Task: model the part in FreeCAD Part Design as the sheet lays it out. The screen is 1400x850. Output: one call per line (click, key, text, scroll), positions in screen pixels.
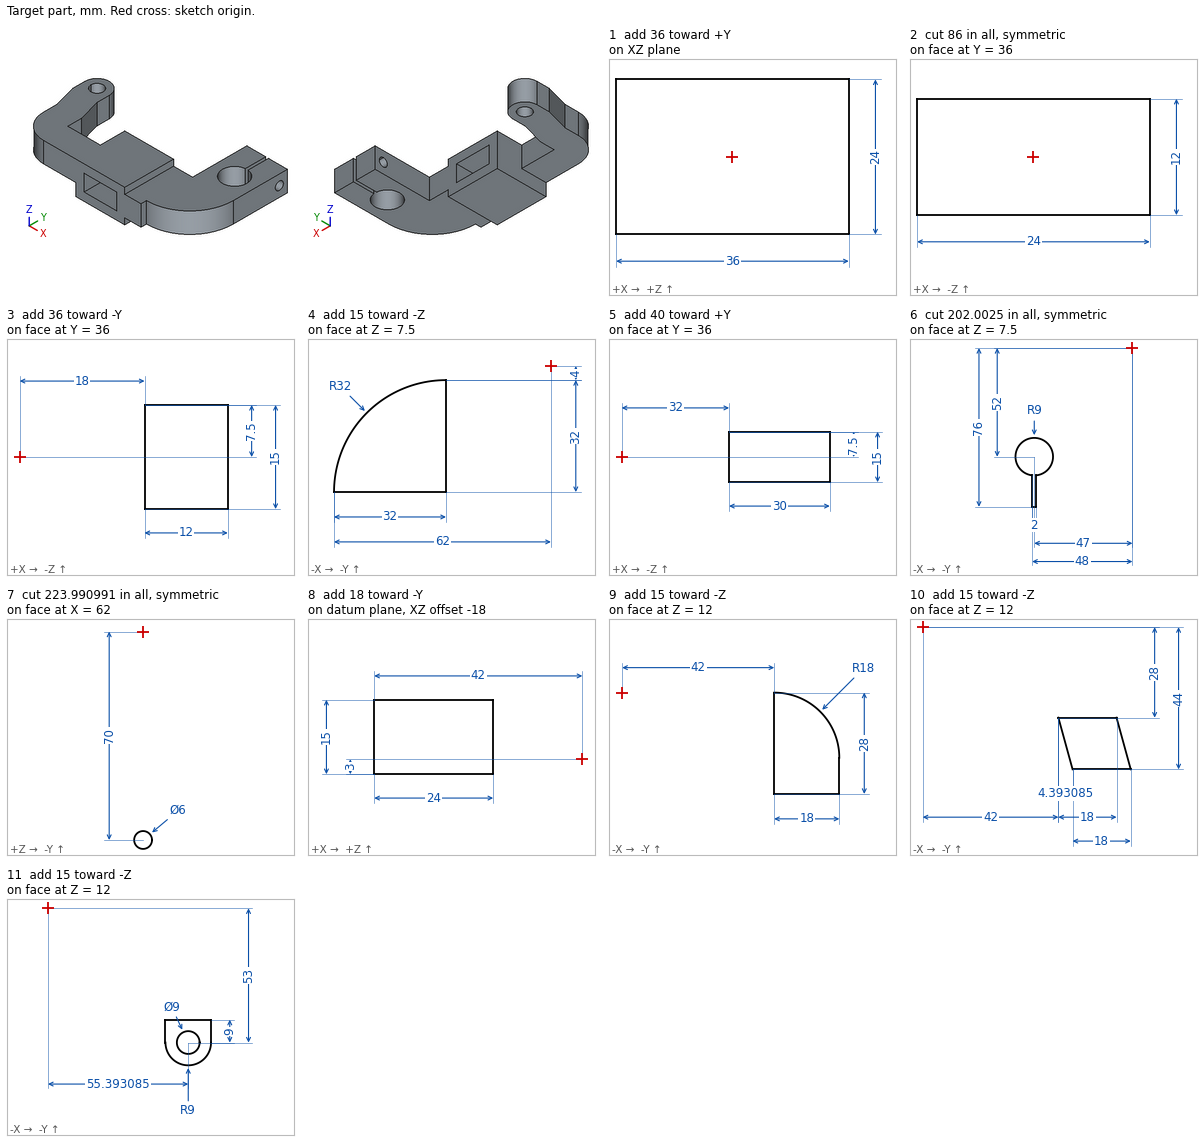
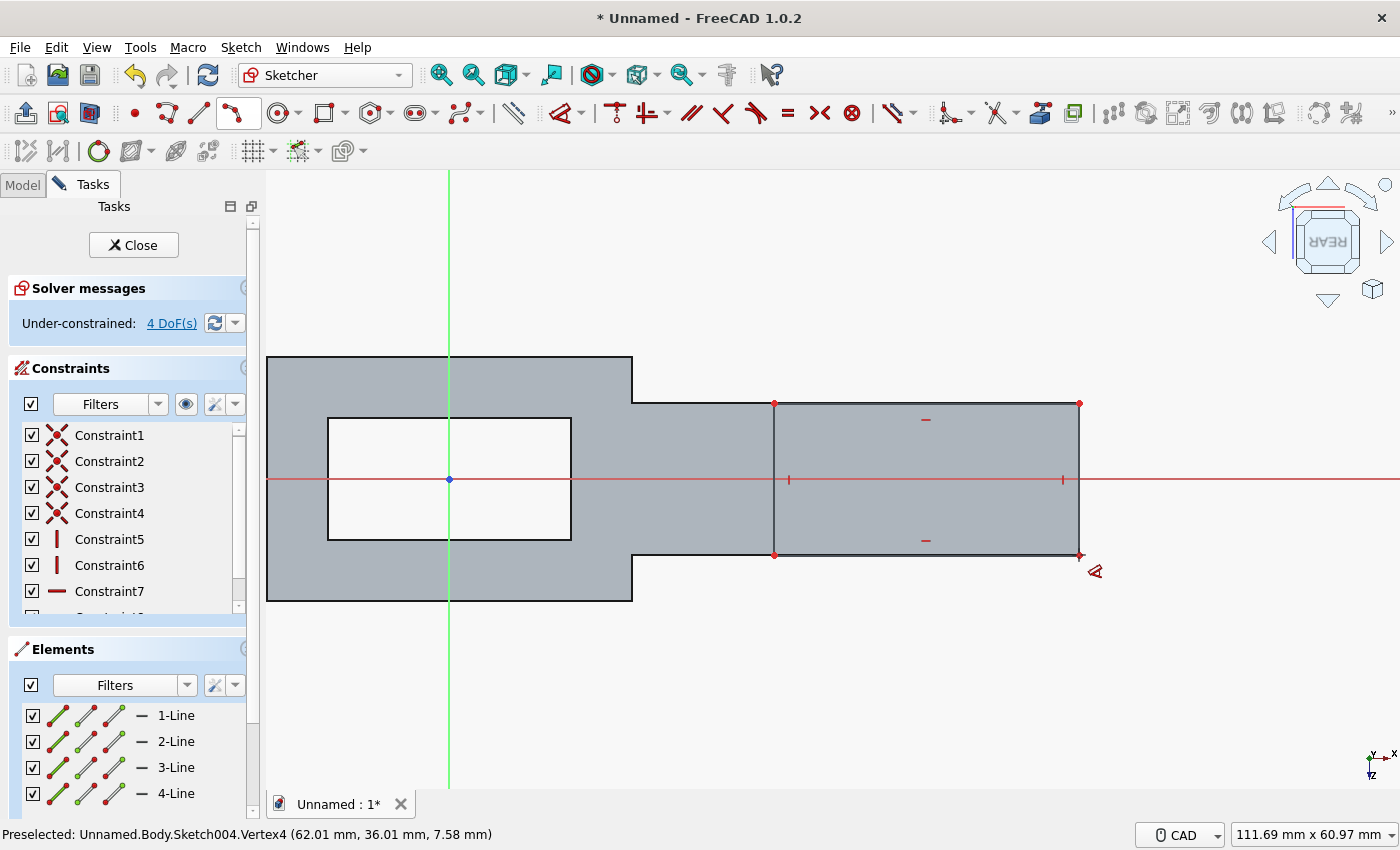
click(774, 450)
click(808, 445)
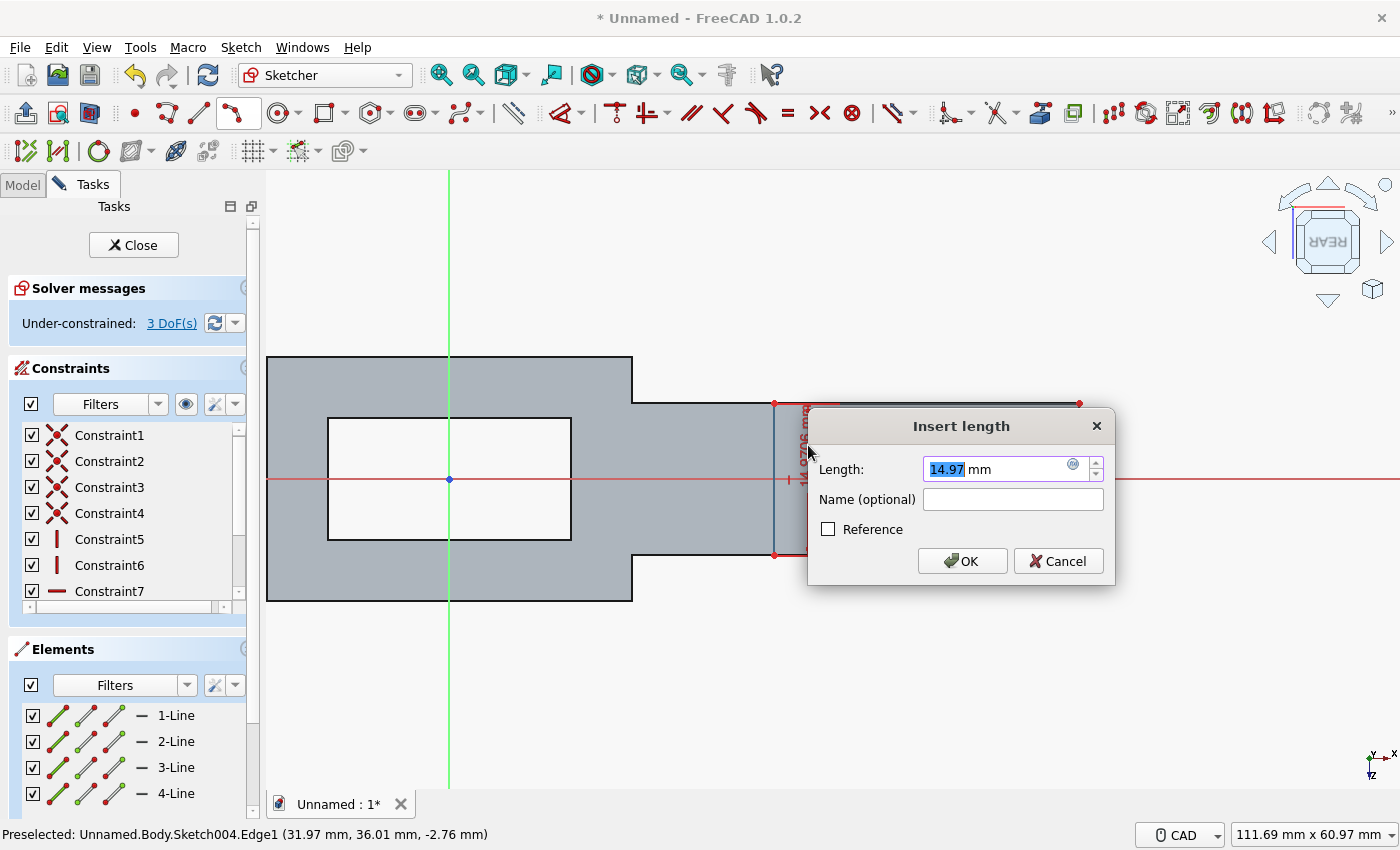
text(15)
key(Return)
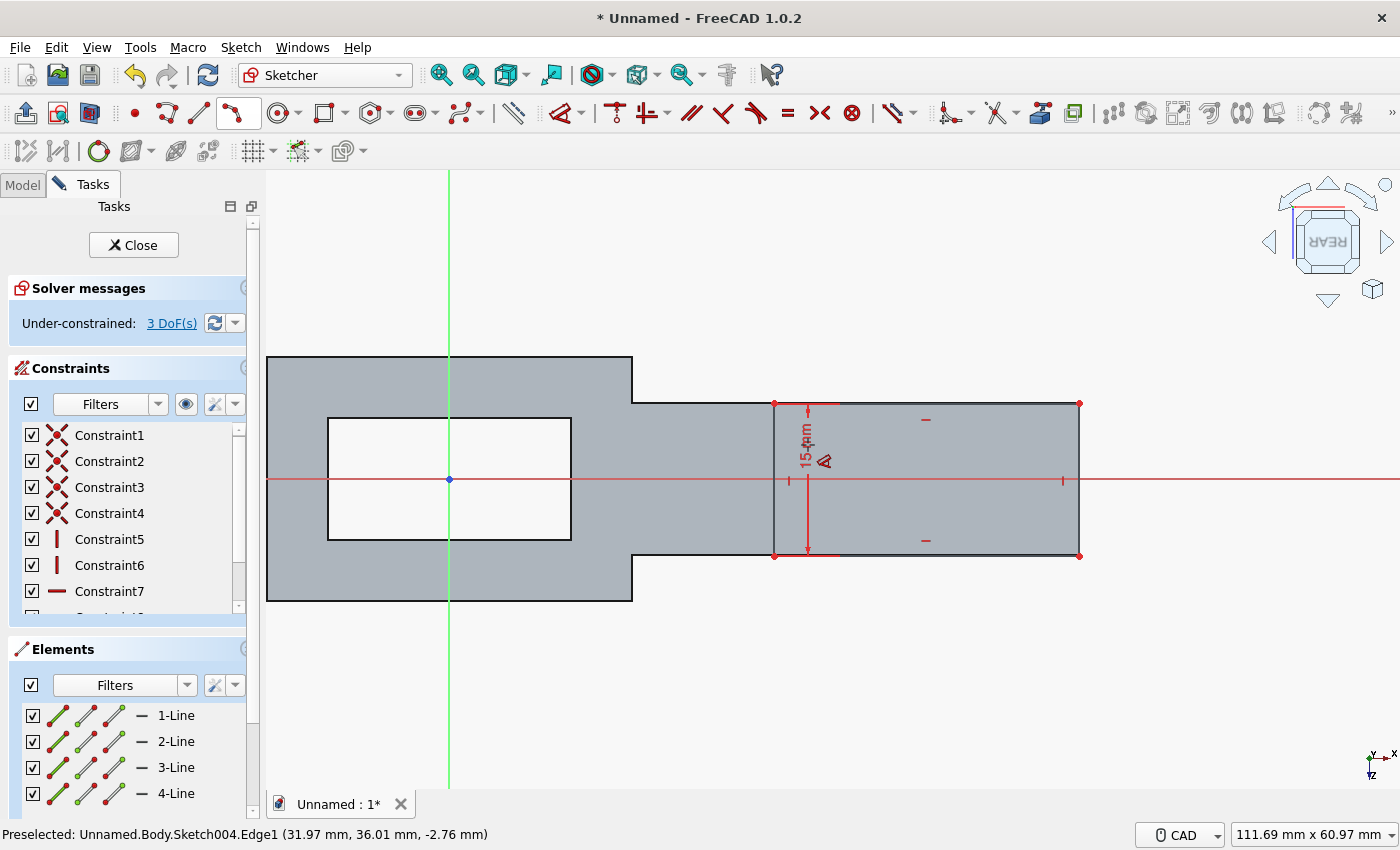
click(866, 556)
click(926, 590)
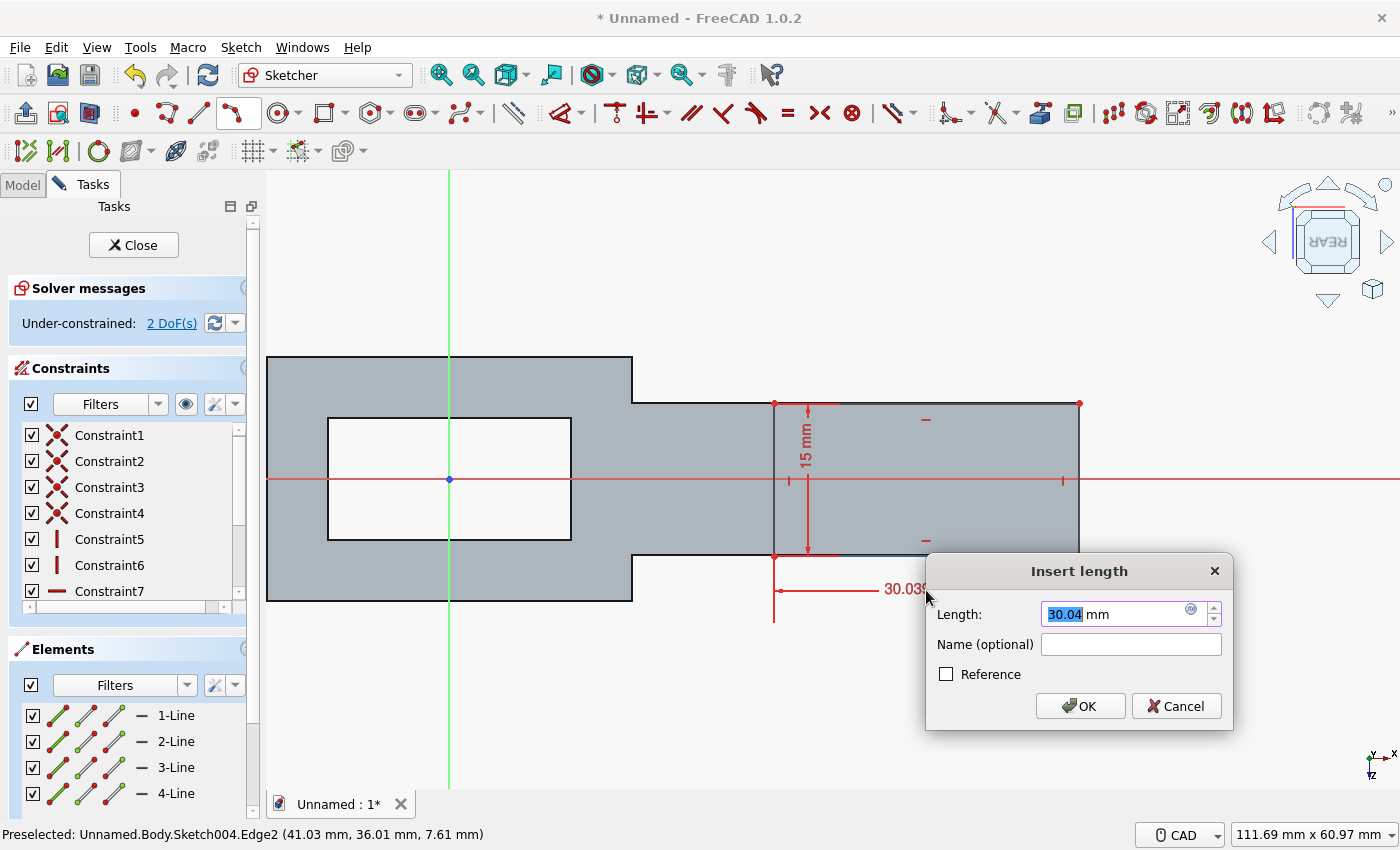
text(30)
key(Return)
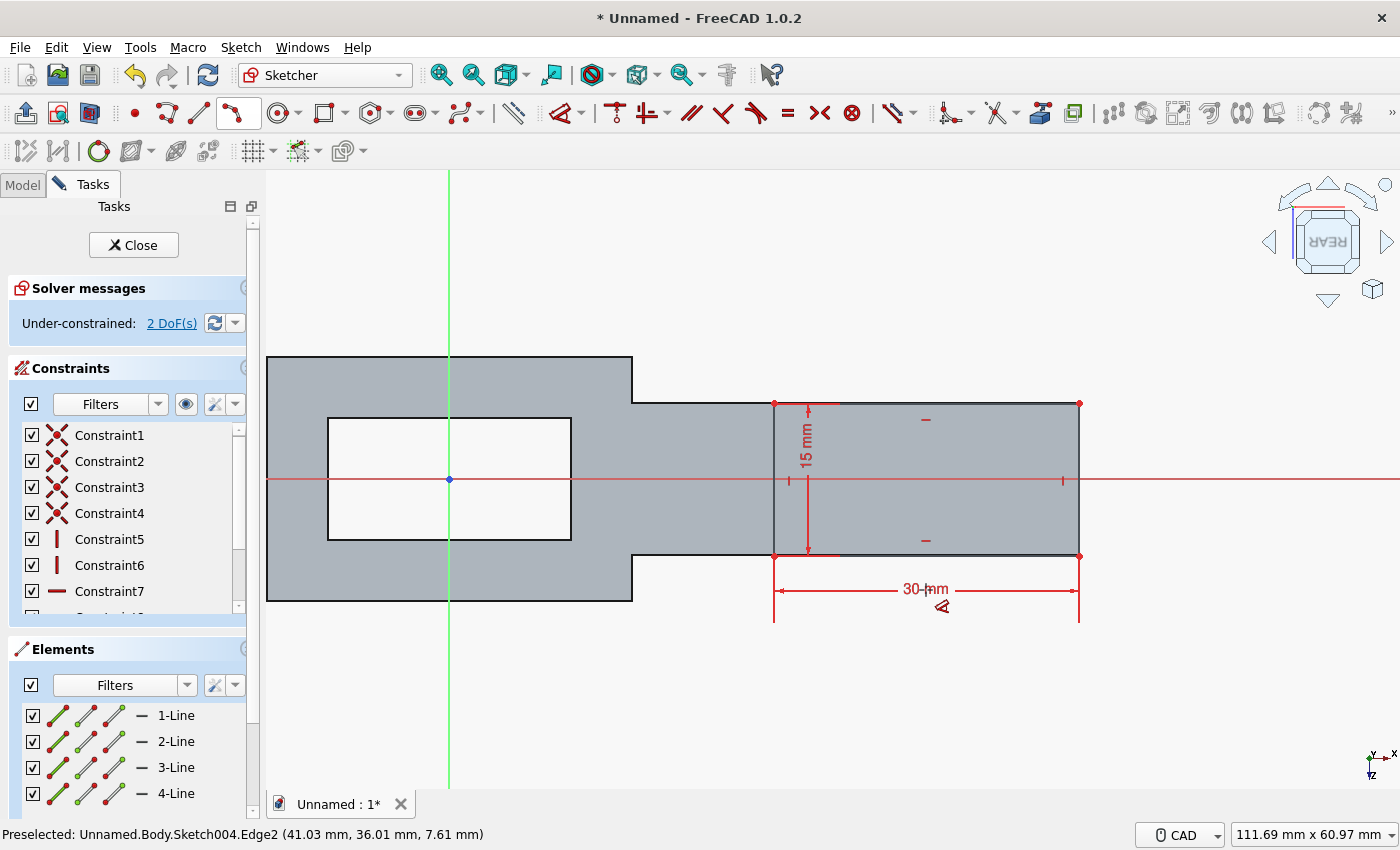
click(774, 404)
click(612, 370)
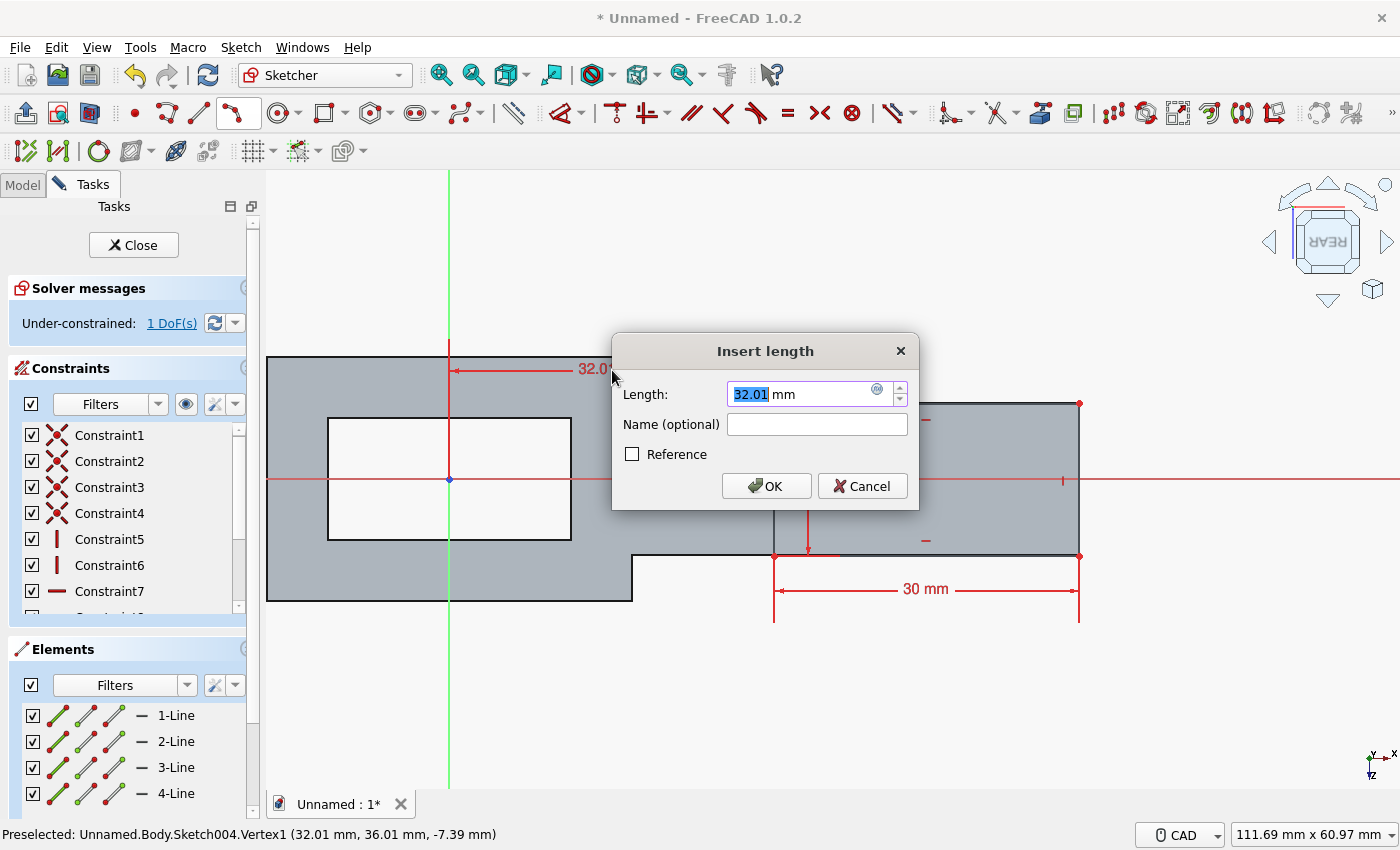
text(32)
key(Return)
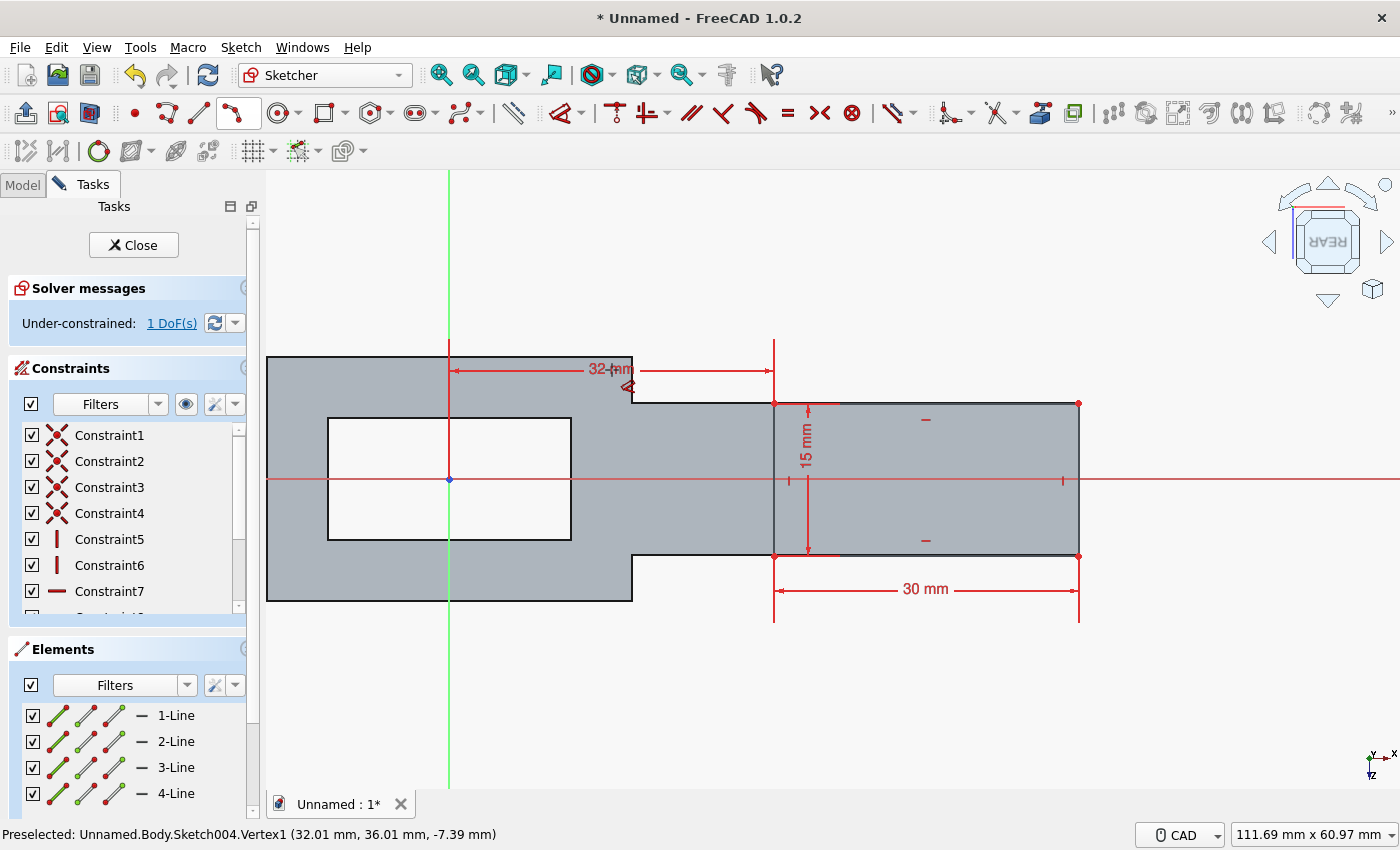
click(774, 404)
click(415, 442)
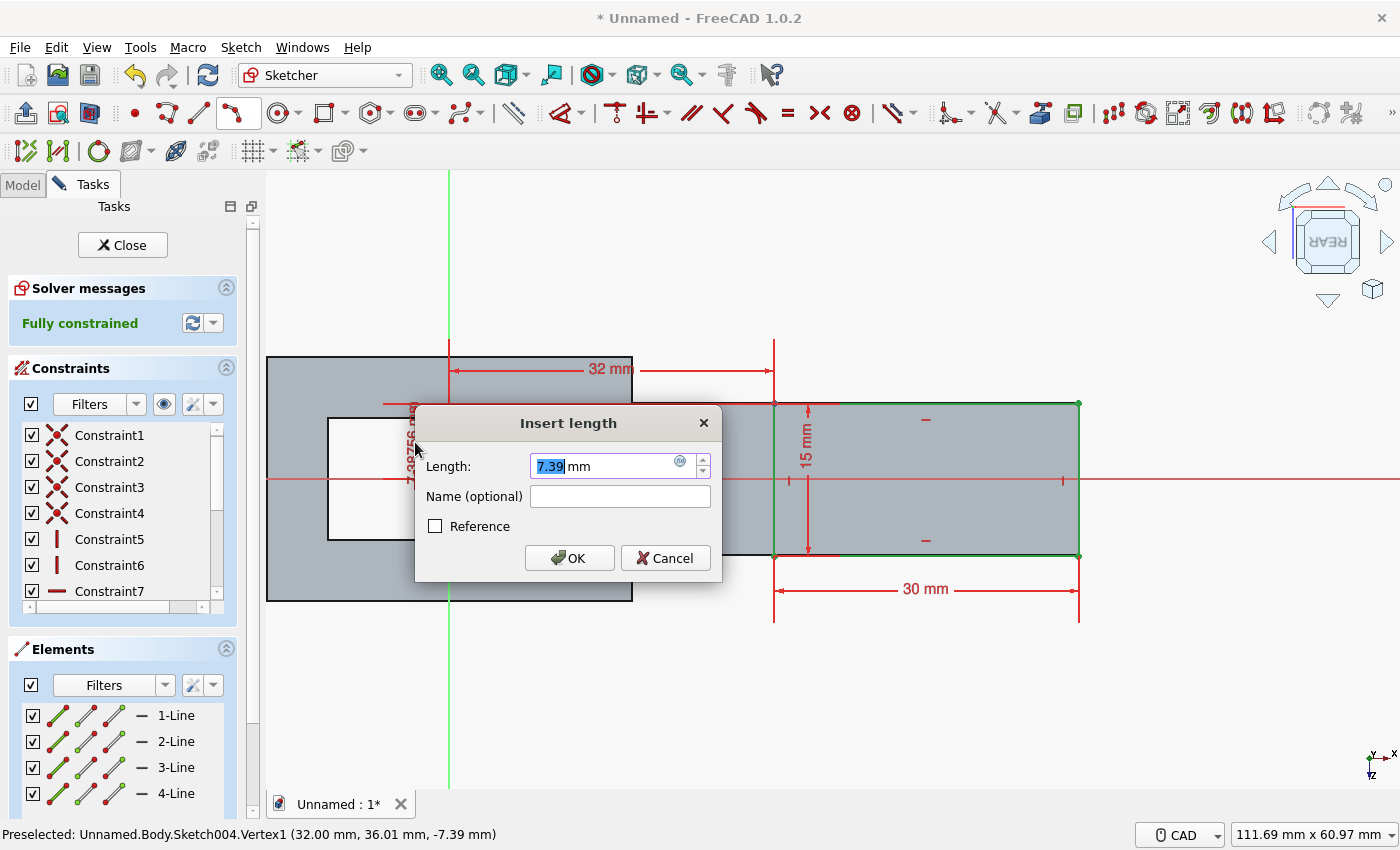
text(7.5)
key(Return)
key(Escape)